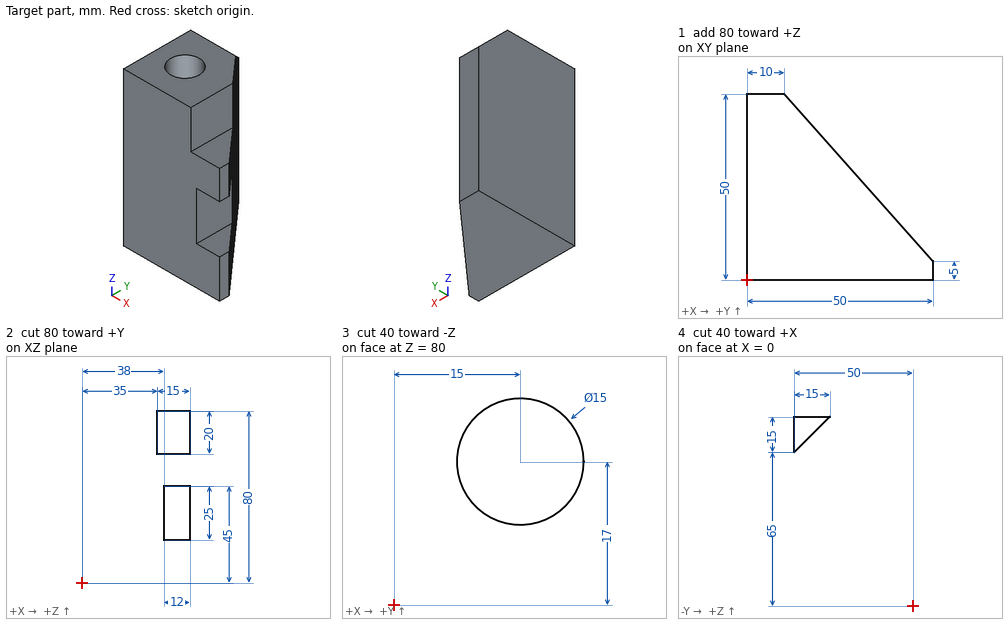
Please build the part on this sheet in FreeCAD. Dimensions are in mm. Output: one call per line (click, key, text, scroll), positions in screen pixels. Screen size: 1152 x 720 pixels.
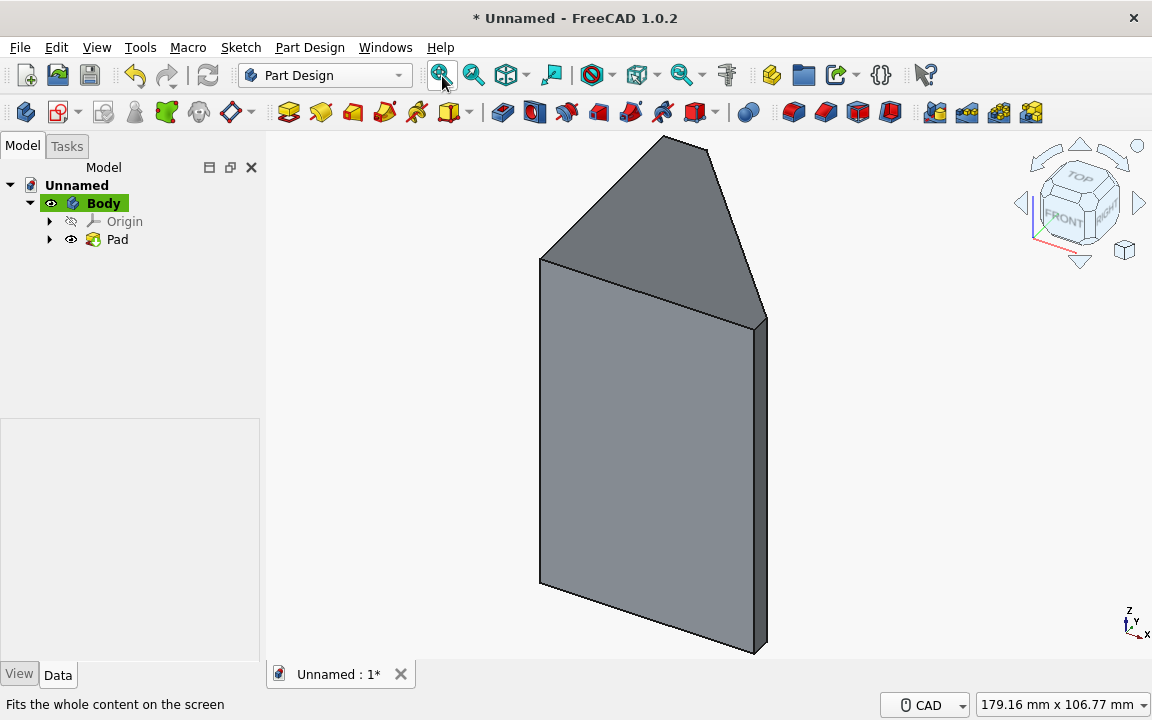
click(58, 112)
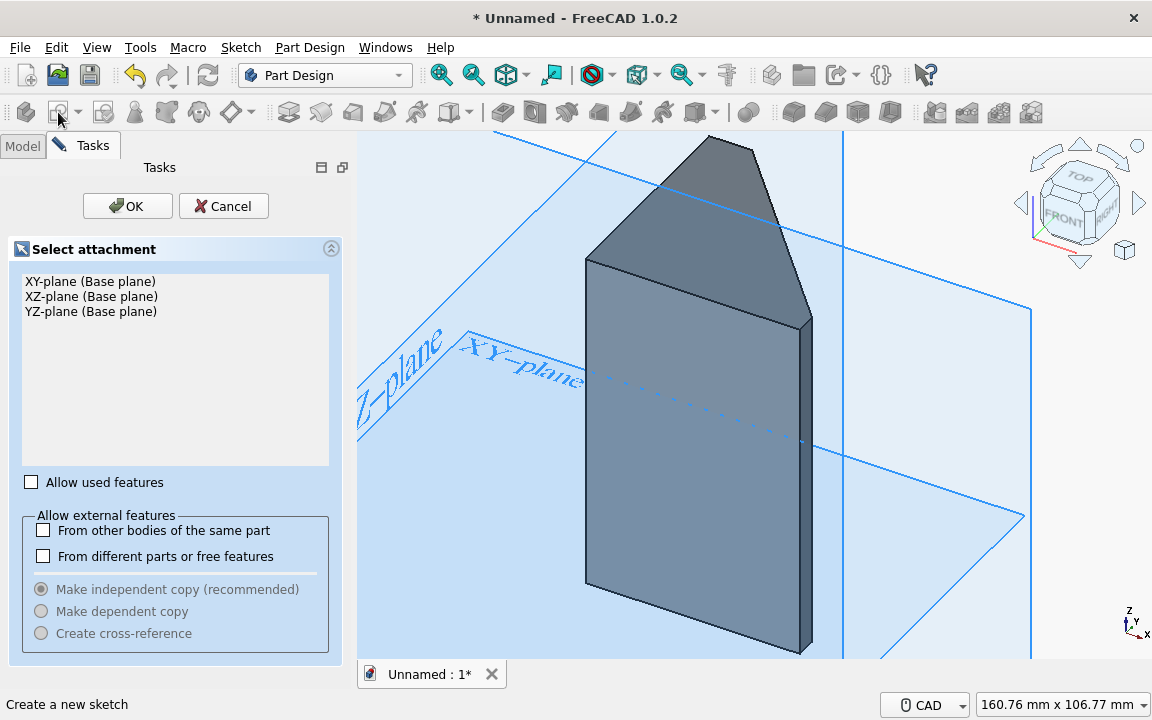
click(82, 296)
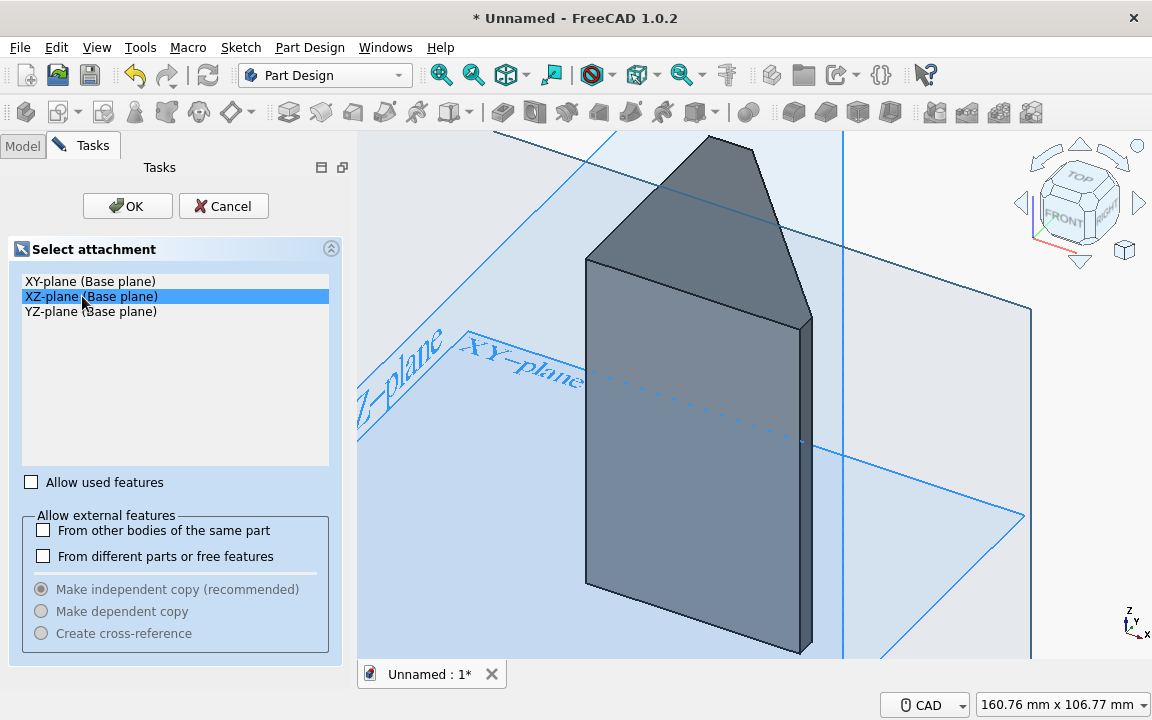
click(128, 206)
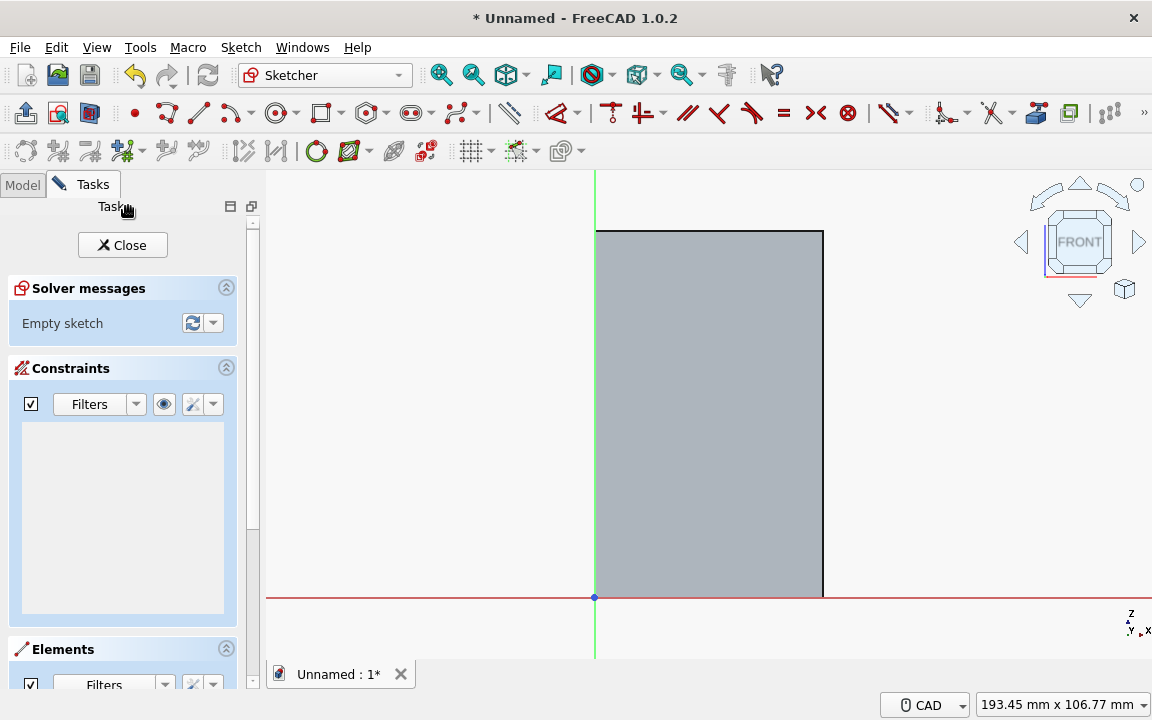
click(322, 114)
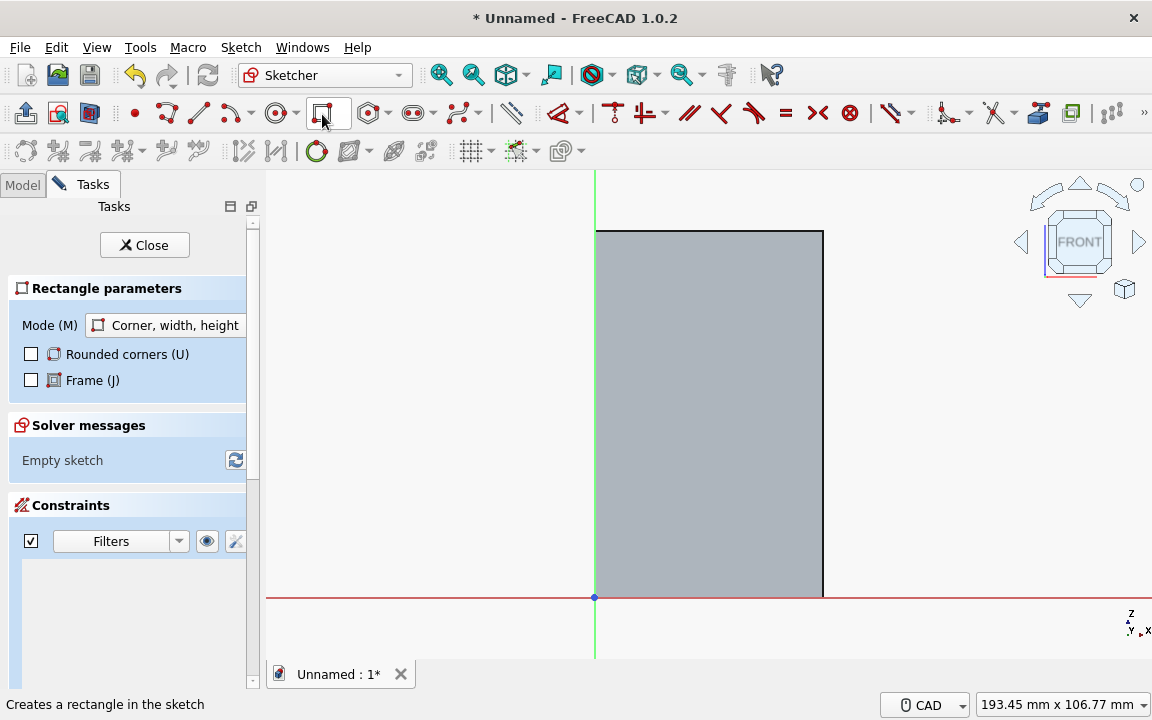
click(755, 231)
click(823, 323)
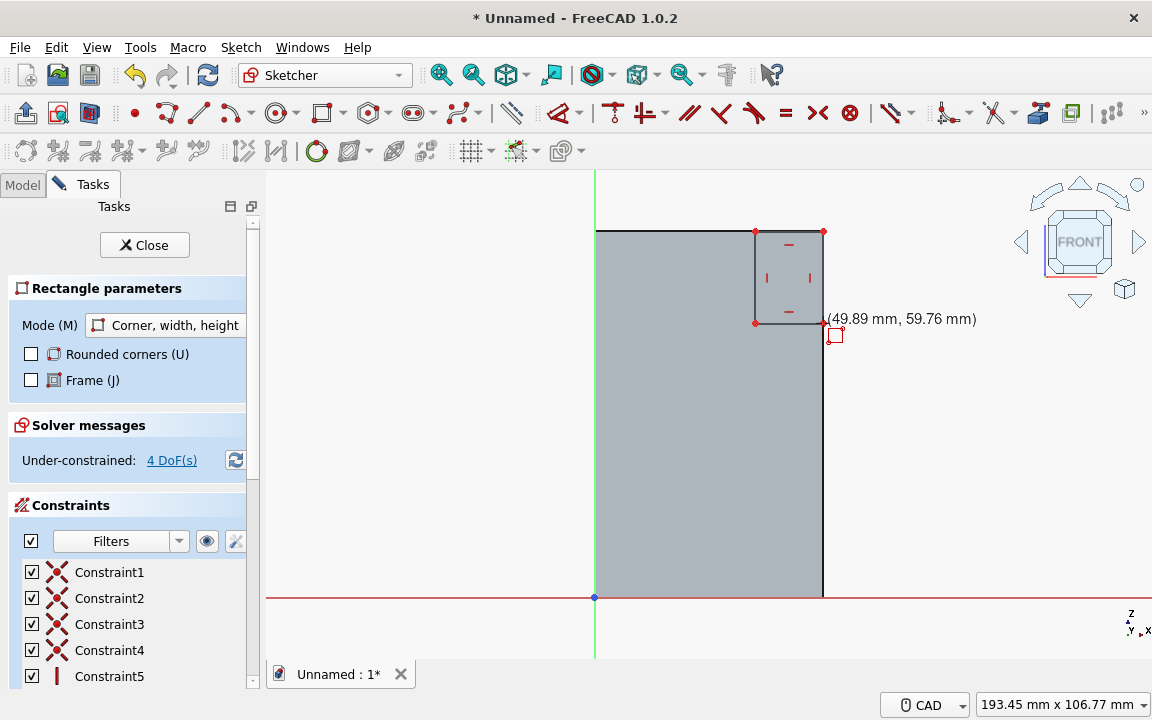
click(769, 392)
click(823, 506)
key(Escape)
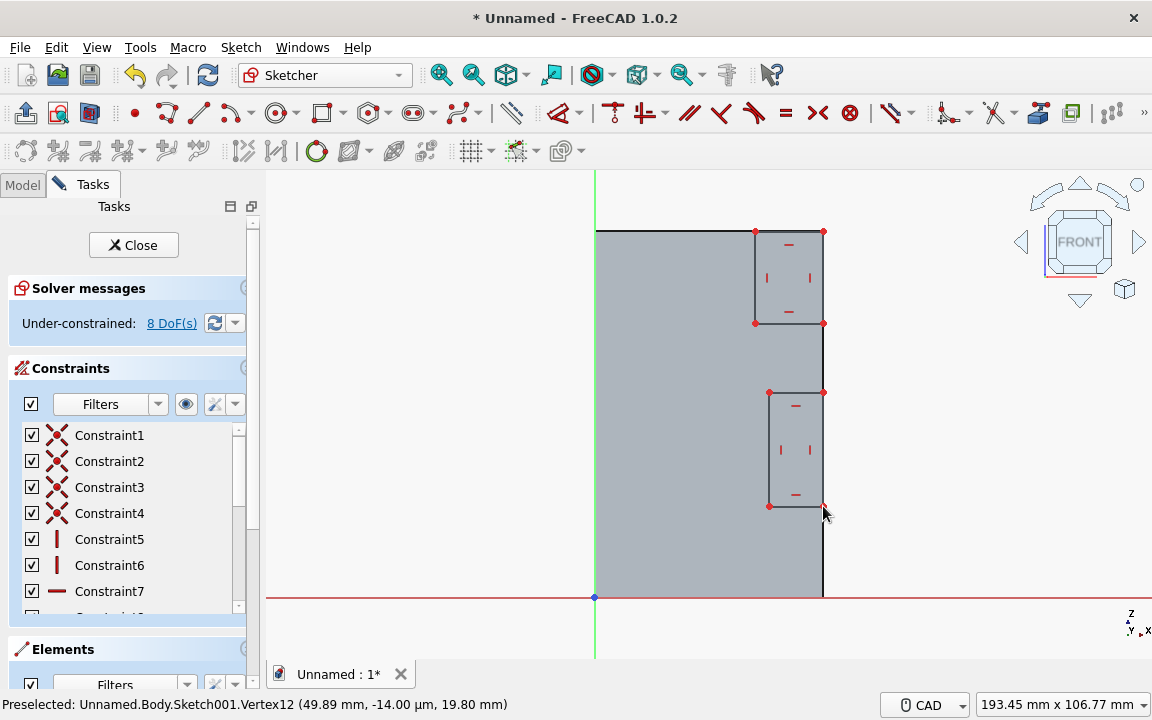
click(558, 114)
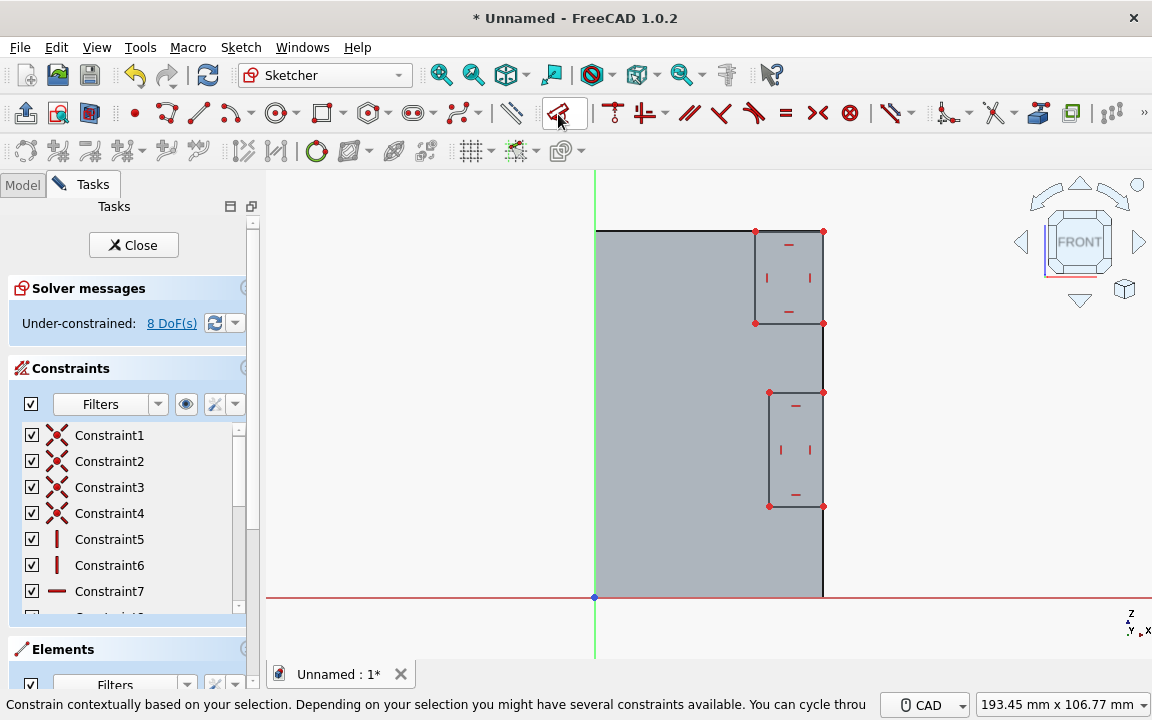
click(755, 260)
click(789, 278)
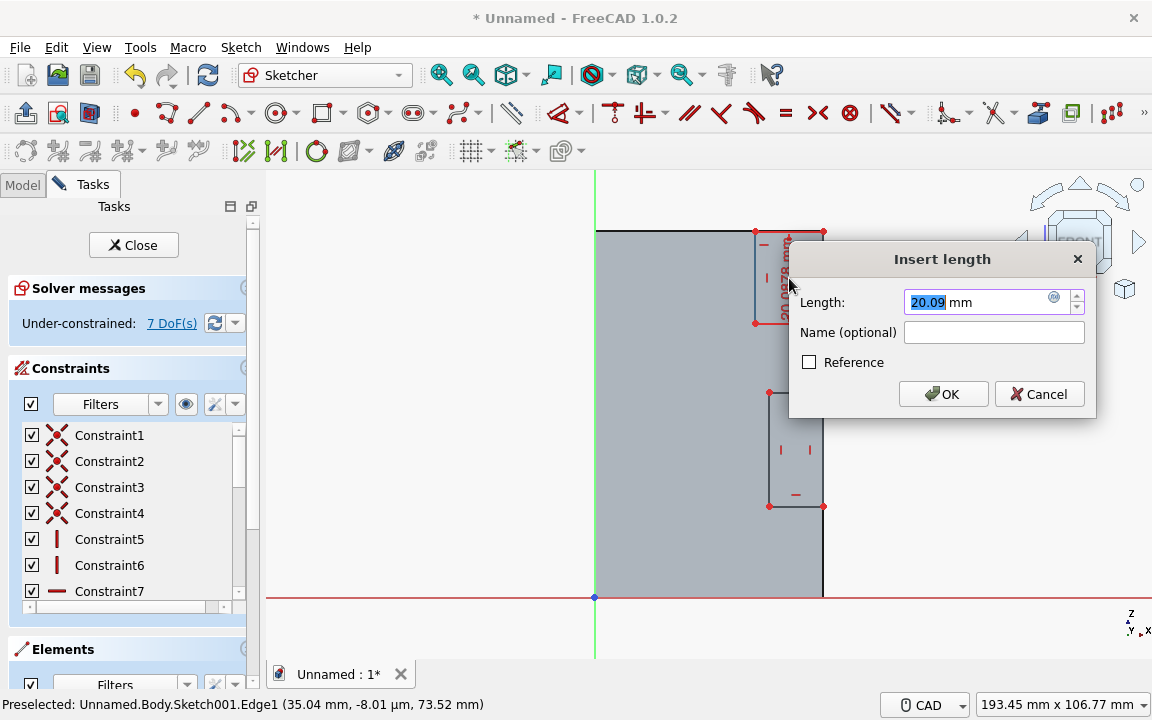
text(20)
key(Return)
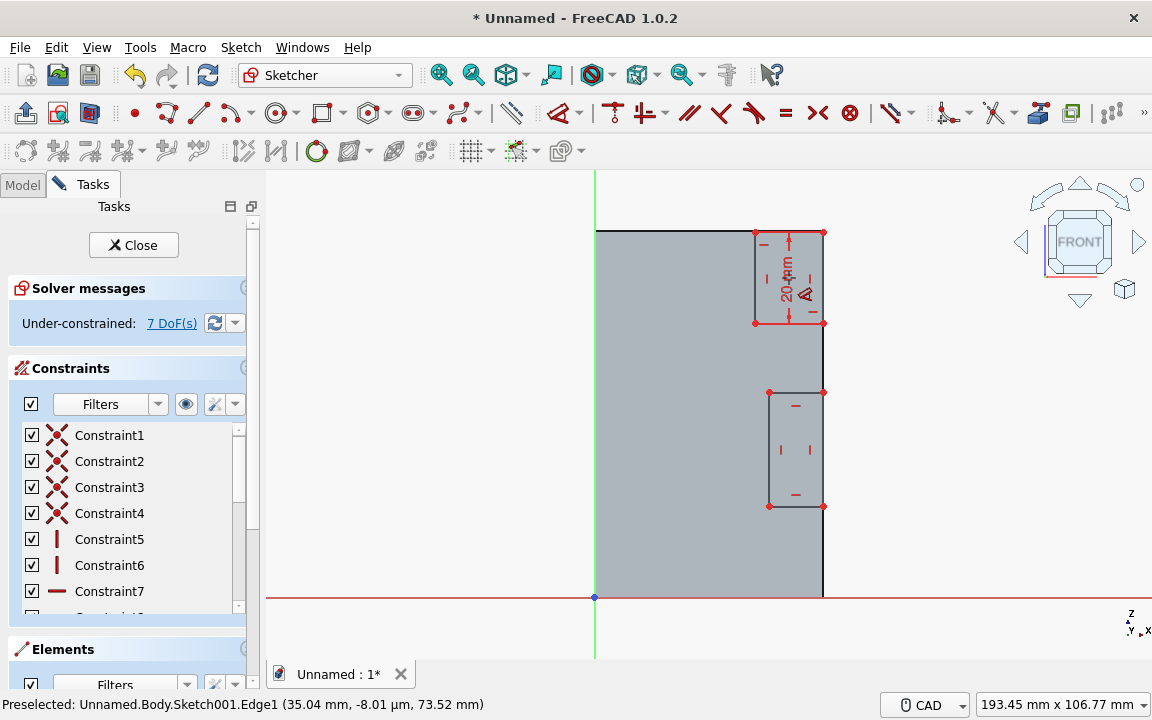
click(775, 324)
click(789, 358)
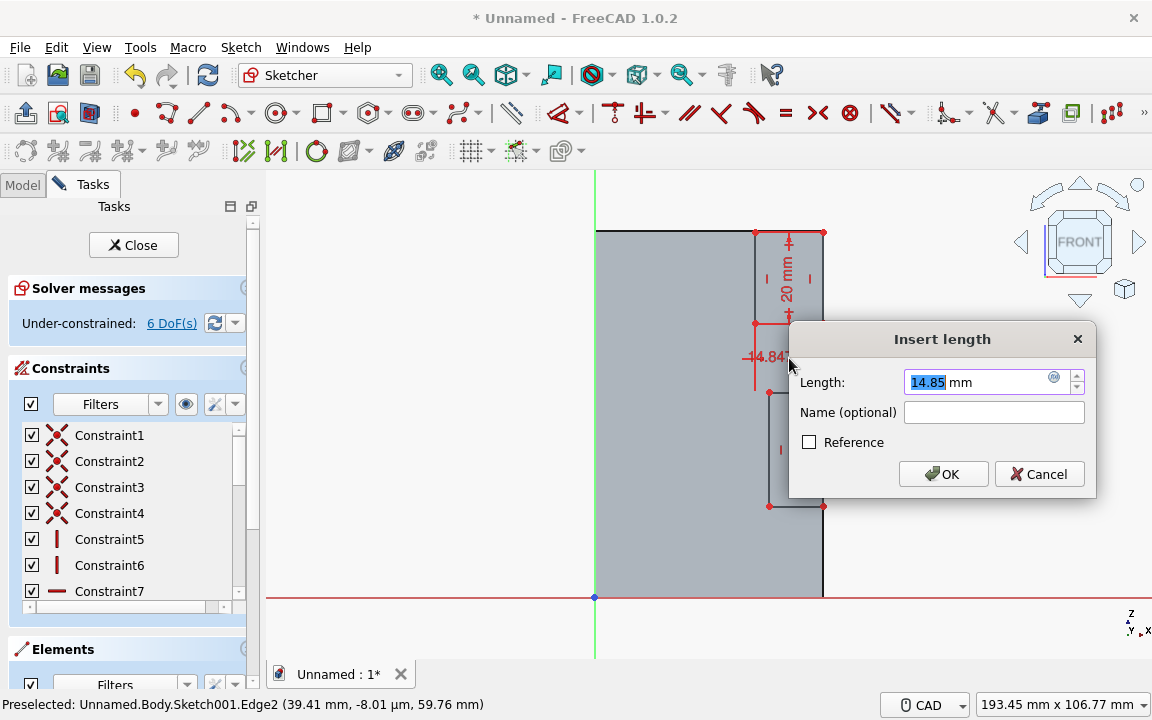
text(15)
key(Return)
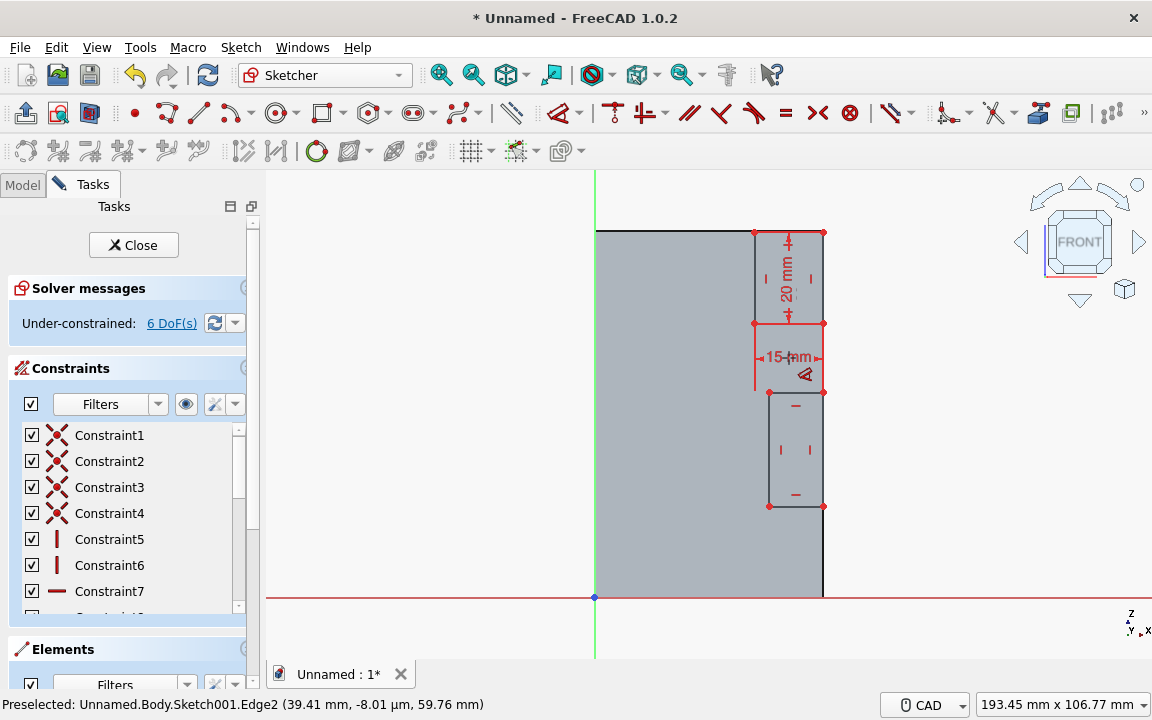
click(769, 427)
click(803, 450)